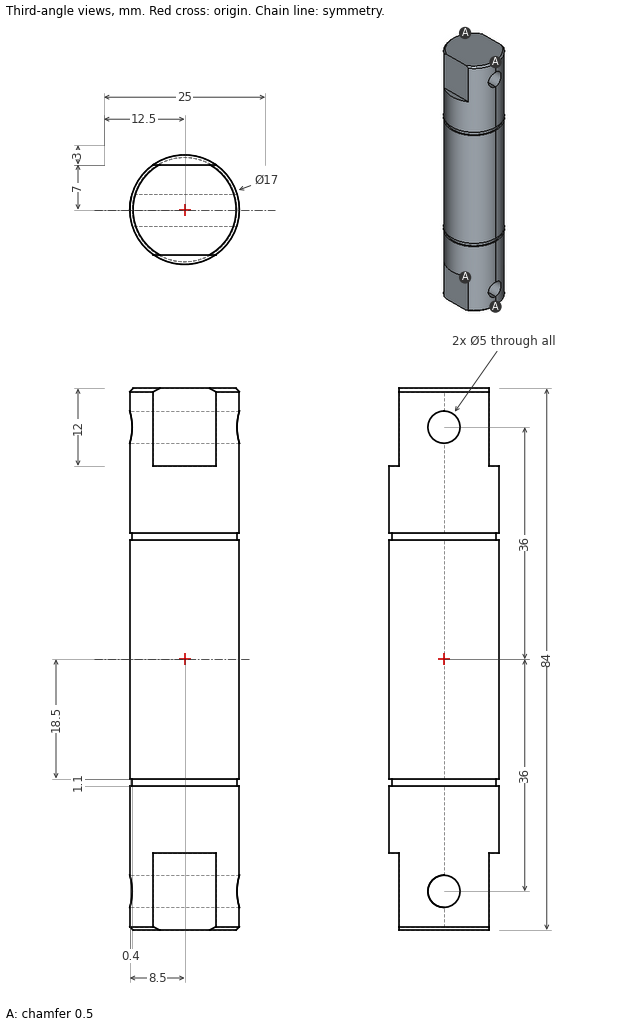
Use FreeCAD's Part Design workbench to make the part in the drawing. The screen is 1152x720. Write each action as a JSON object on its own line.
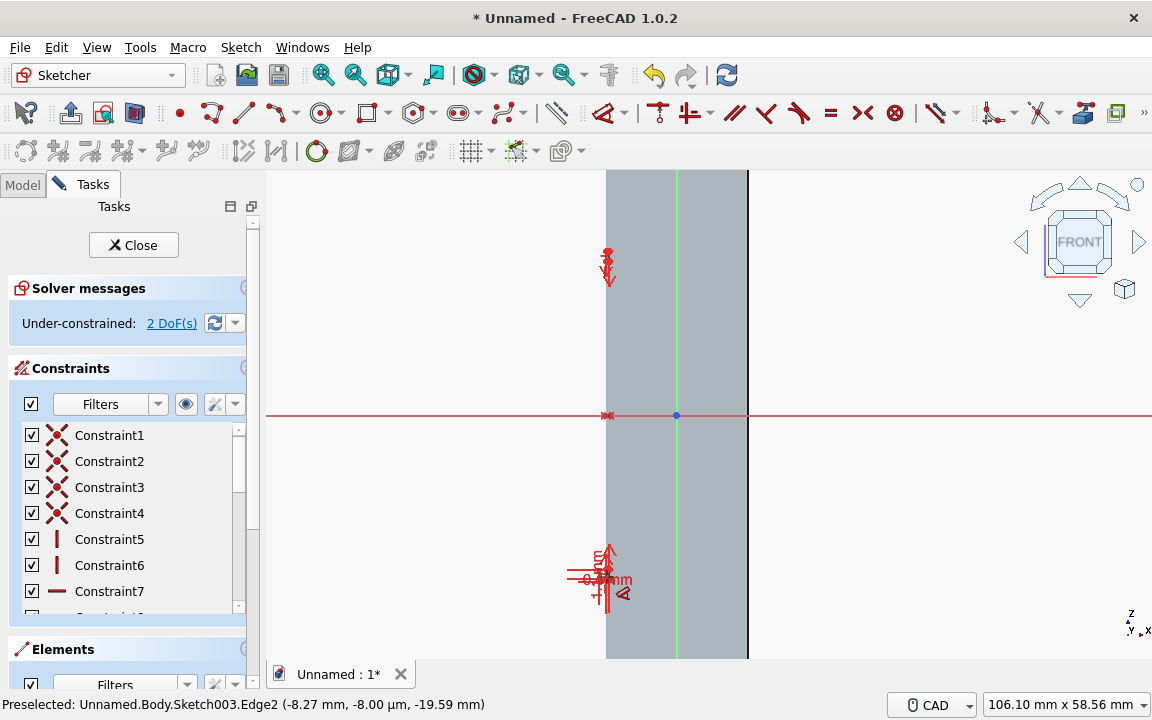
{"action": "scroll", "coordinate": [606, 570], "scroll_direction": "up", "scroll_amount": 7}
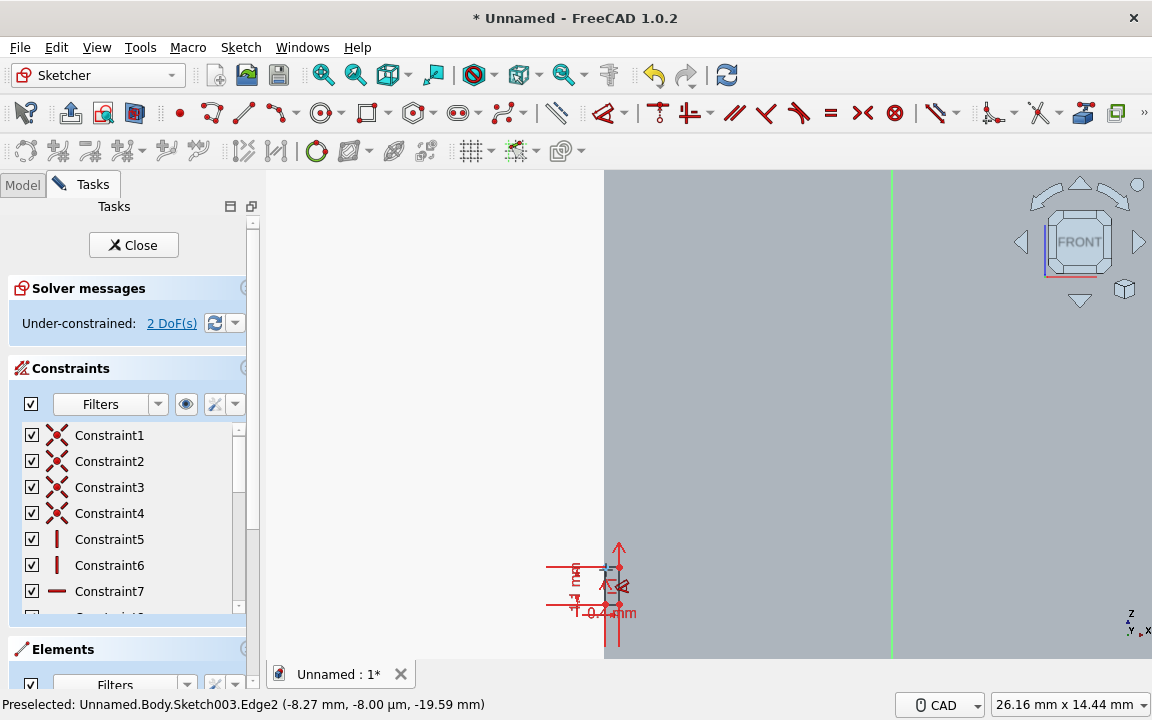
{"action": "left_click", "coordinate": [605, 567]}
{"action": "left_click", "coordinate": [749, 601]}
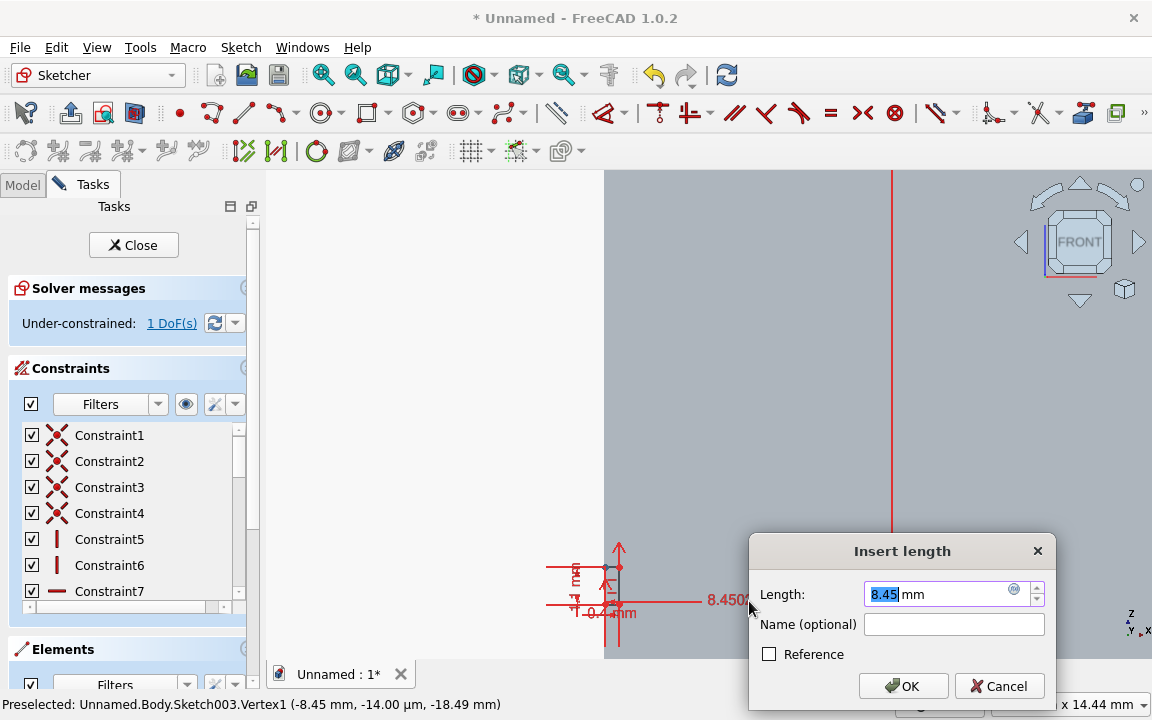
{"action": "type", "text": "8.5"}
{"action": "key", "text": "Return"}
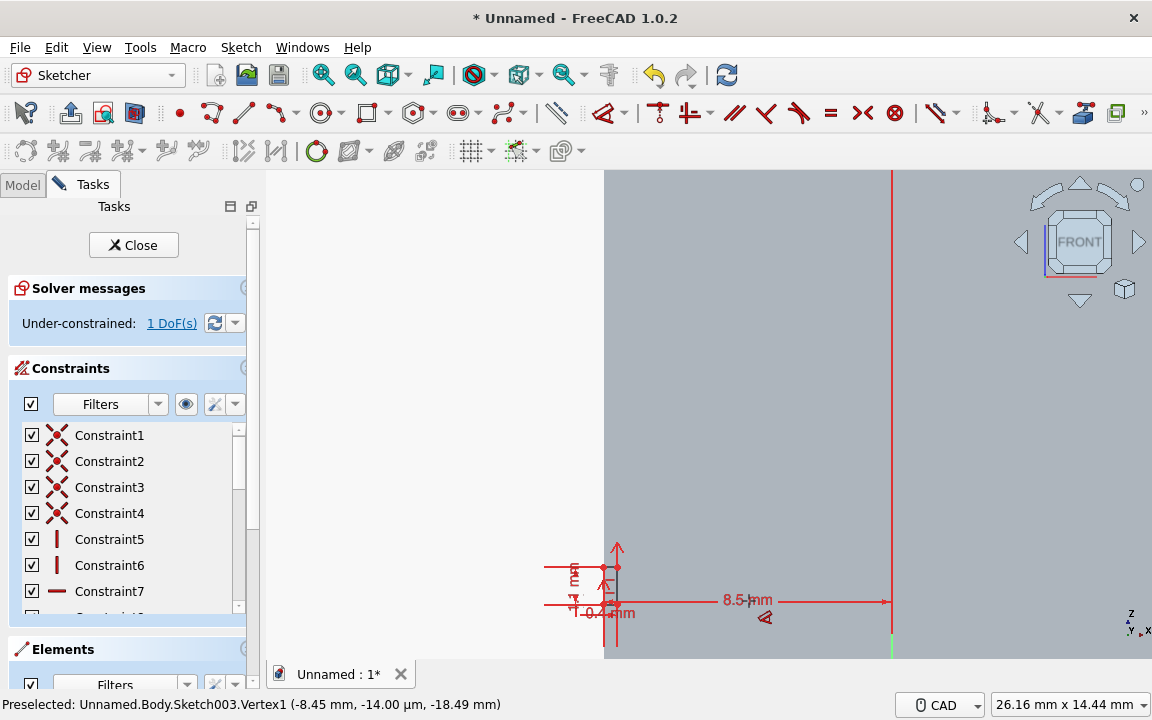
{"action": "left_click", "coordinate": [604, 567]}
{"action": "left_click", "coordinate": [926, 383]}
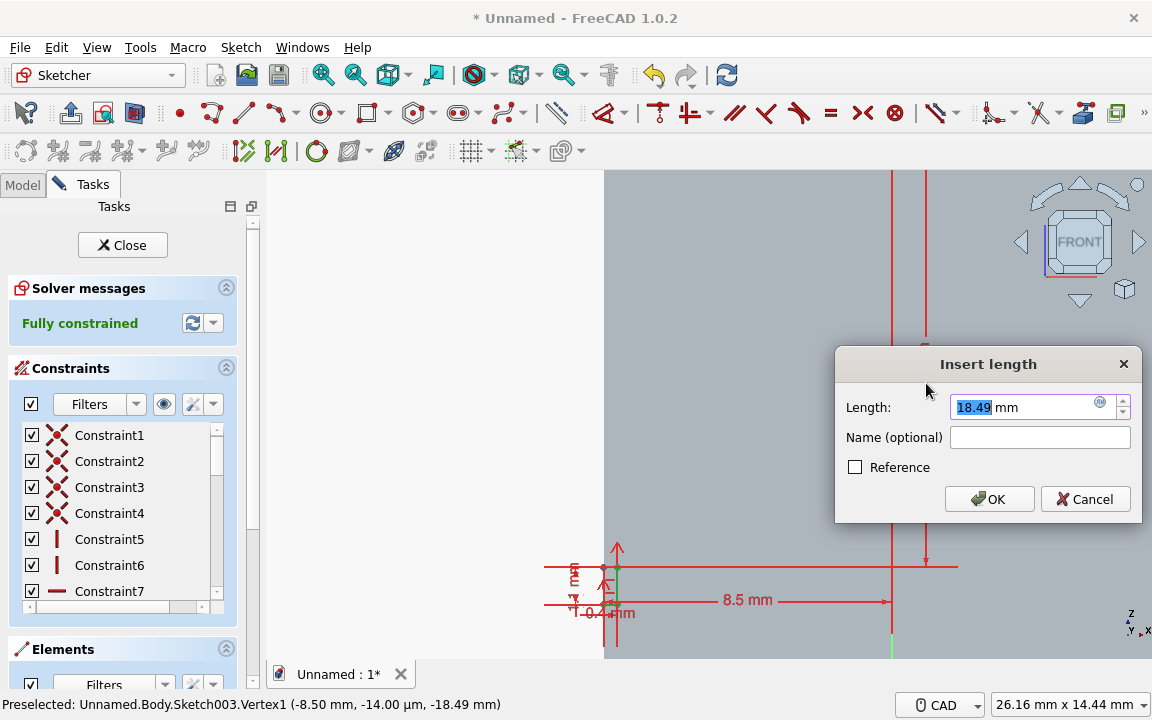
{"action": "type", "text": "18.5"}
{"action": "key", "text": "Return"}
{"action": "key", "text": "Escape"}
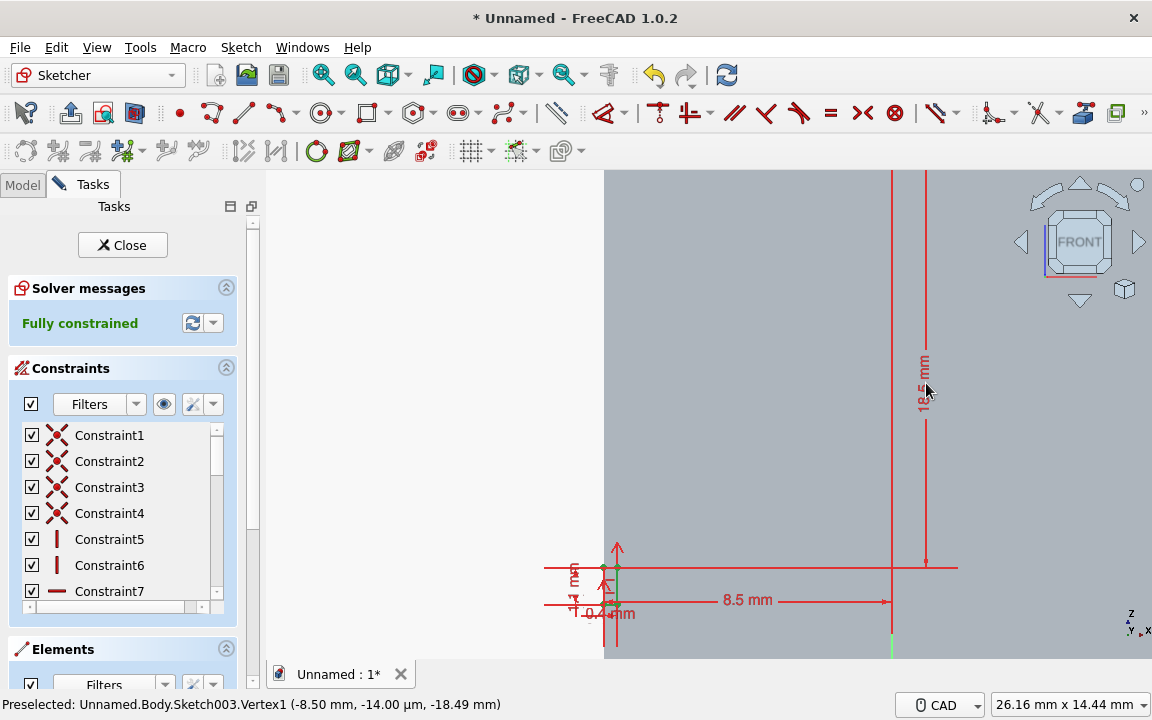
{"action": "left_click", "coordinate": [123, 245]}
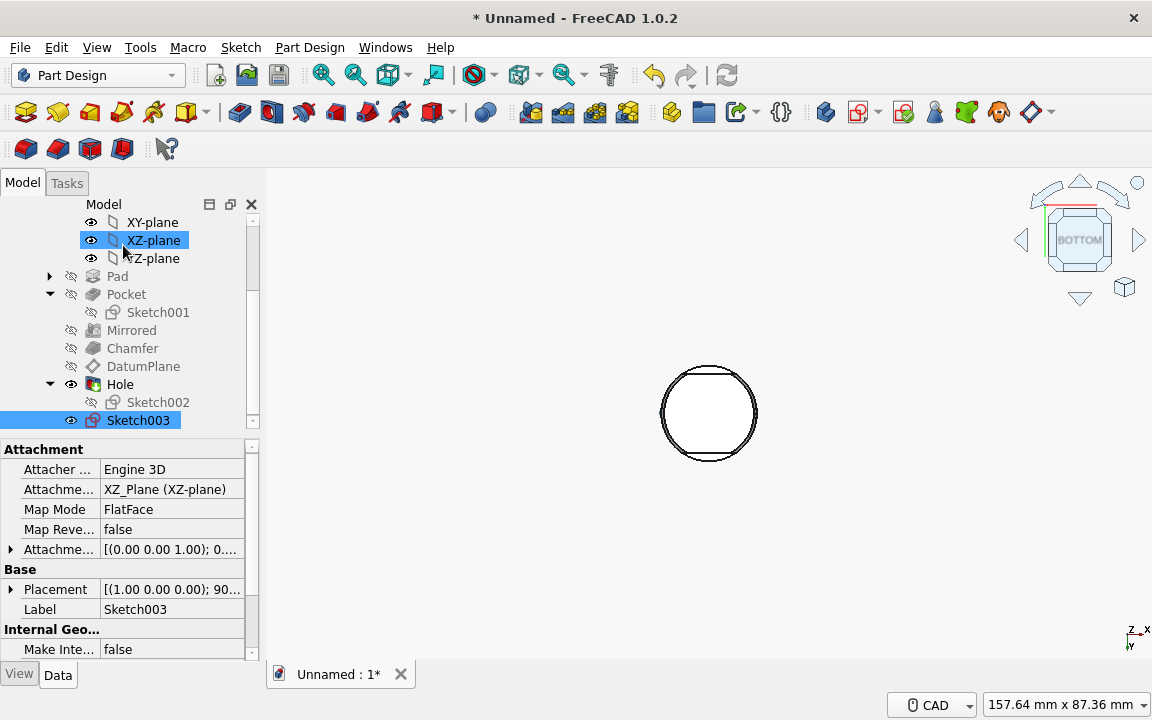
{"action": "left_click", "coordinate": [304, 112]}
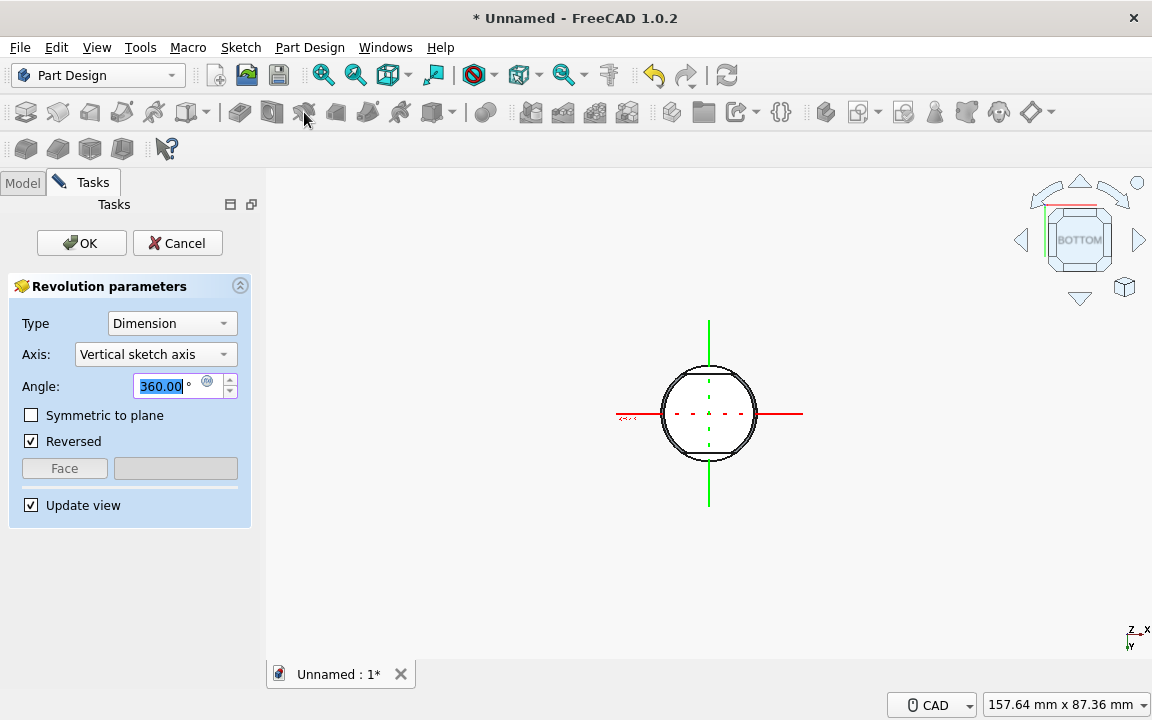
{"action": "left_click", "coordinate": [82, 243]}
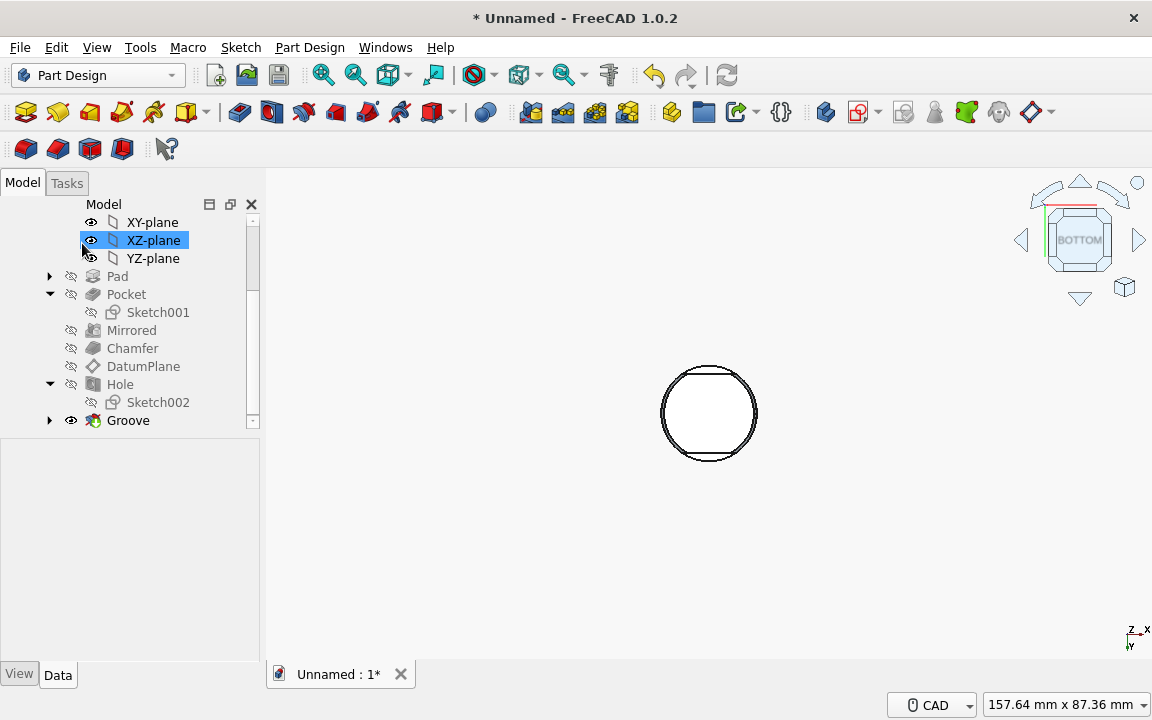
{"action": "key", "text": "0"}